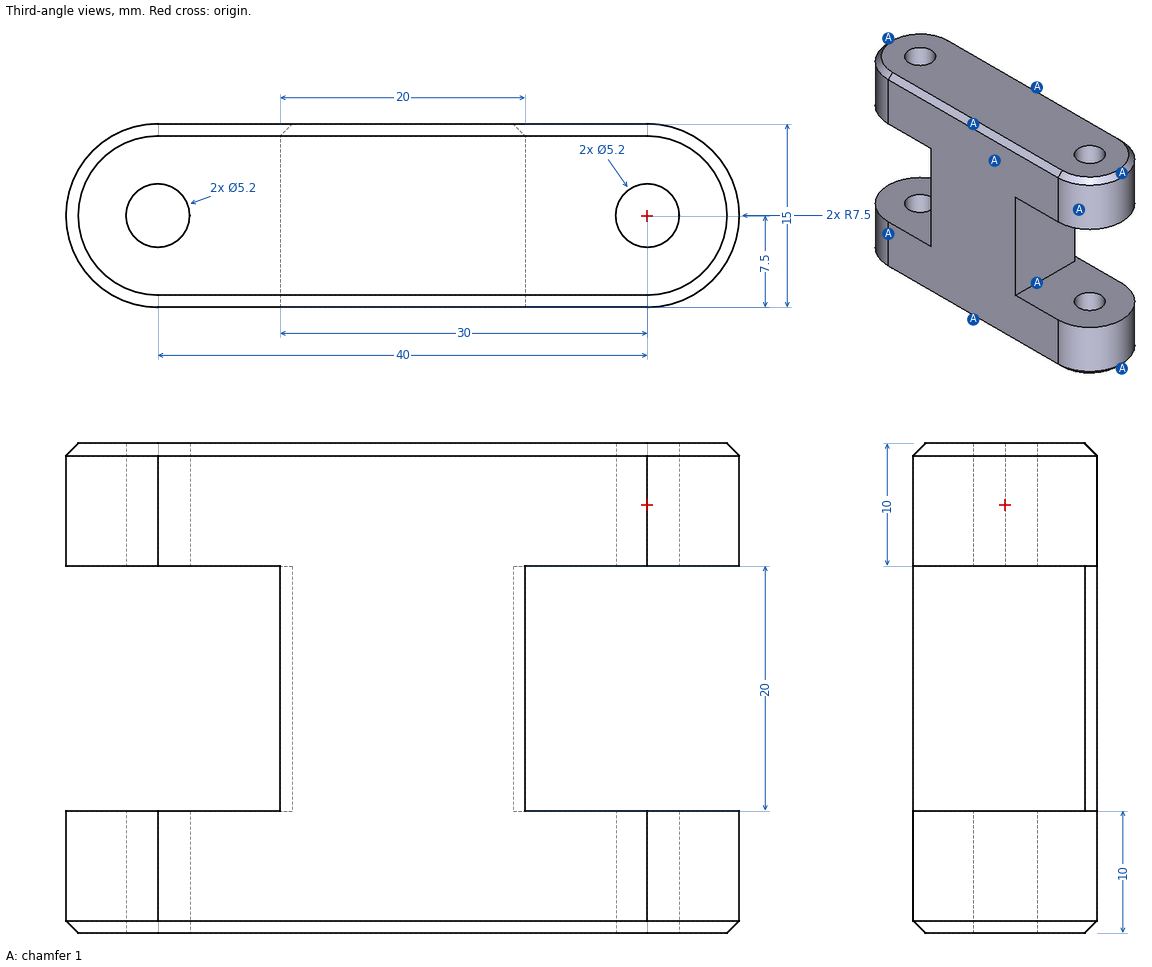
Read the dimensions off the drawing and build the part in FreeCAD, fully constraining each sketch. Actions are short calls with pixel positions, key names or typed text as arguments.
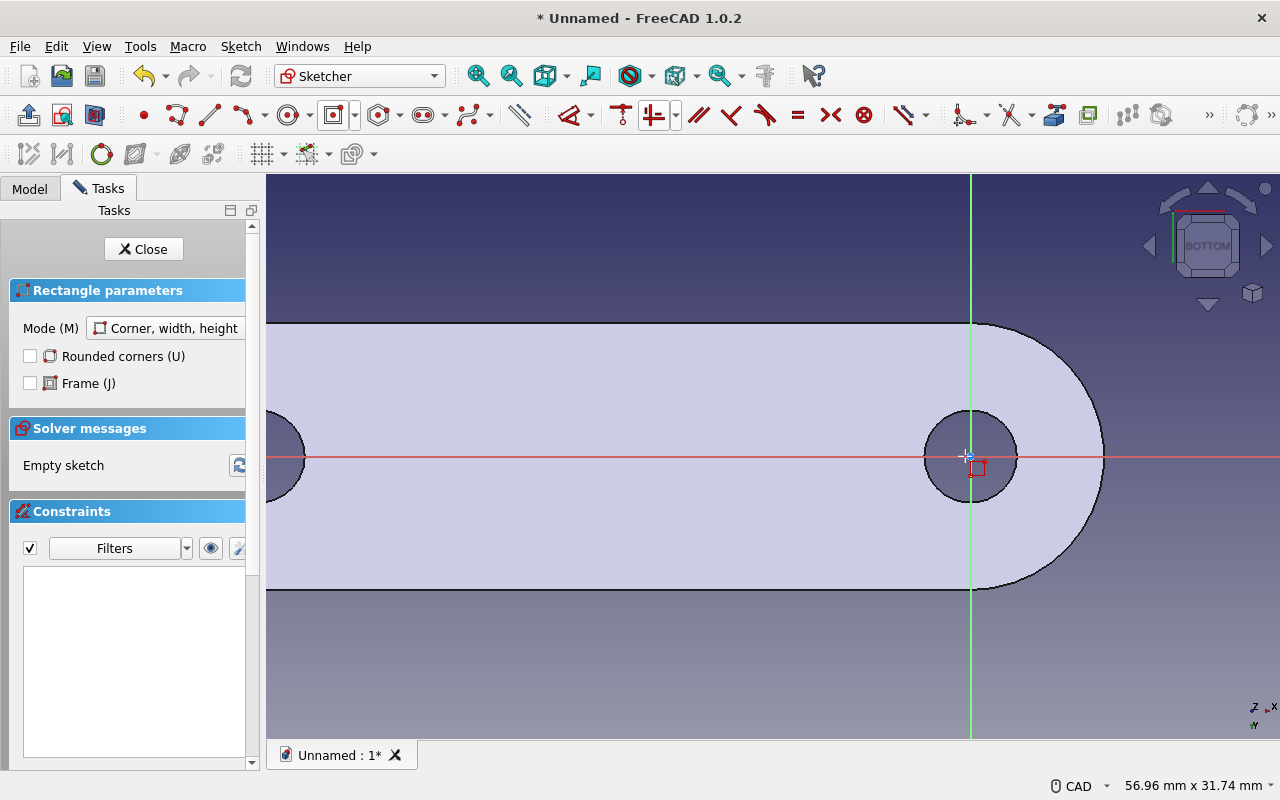
click(437, 323)
move(793, 590)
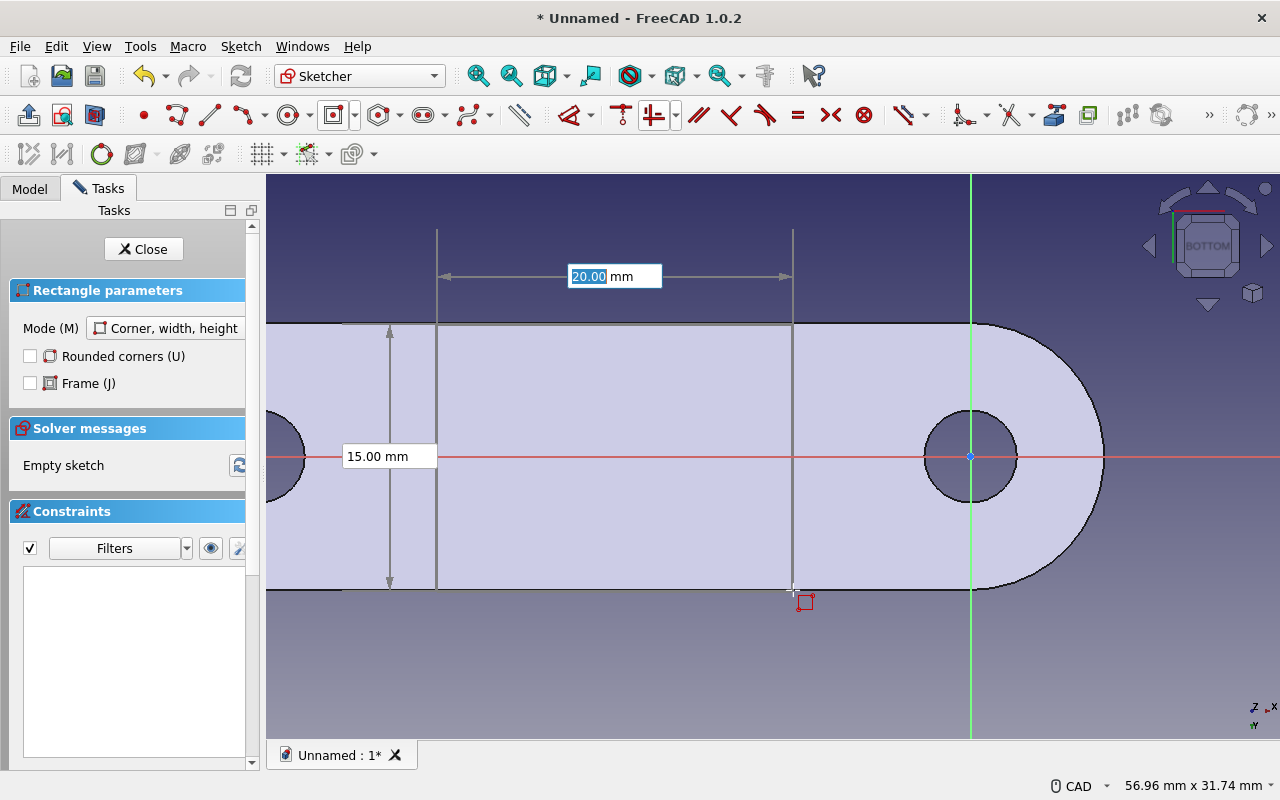
text(20)
key(Tab)
text(15)
key(Return)
key(Escape)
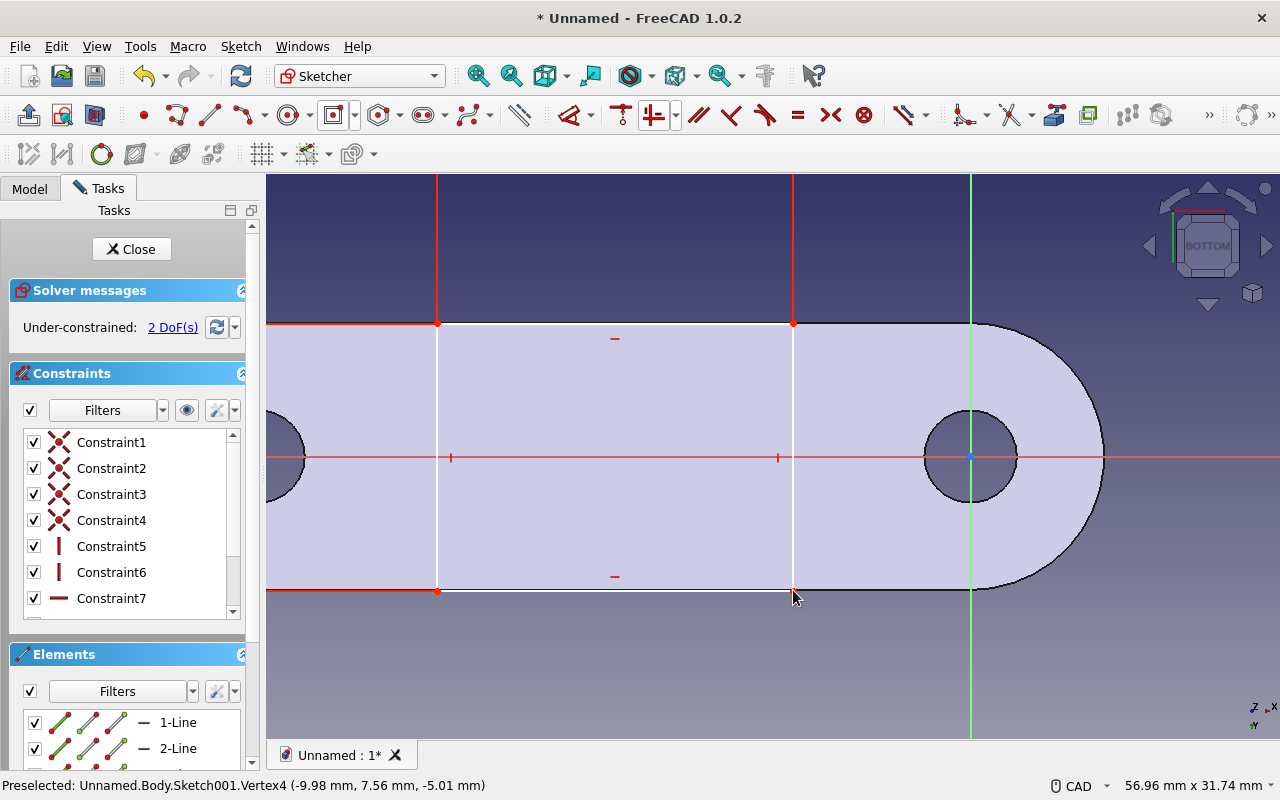
key(d)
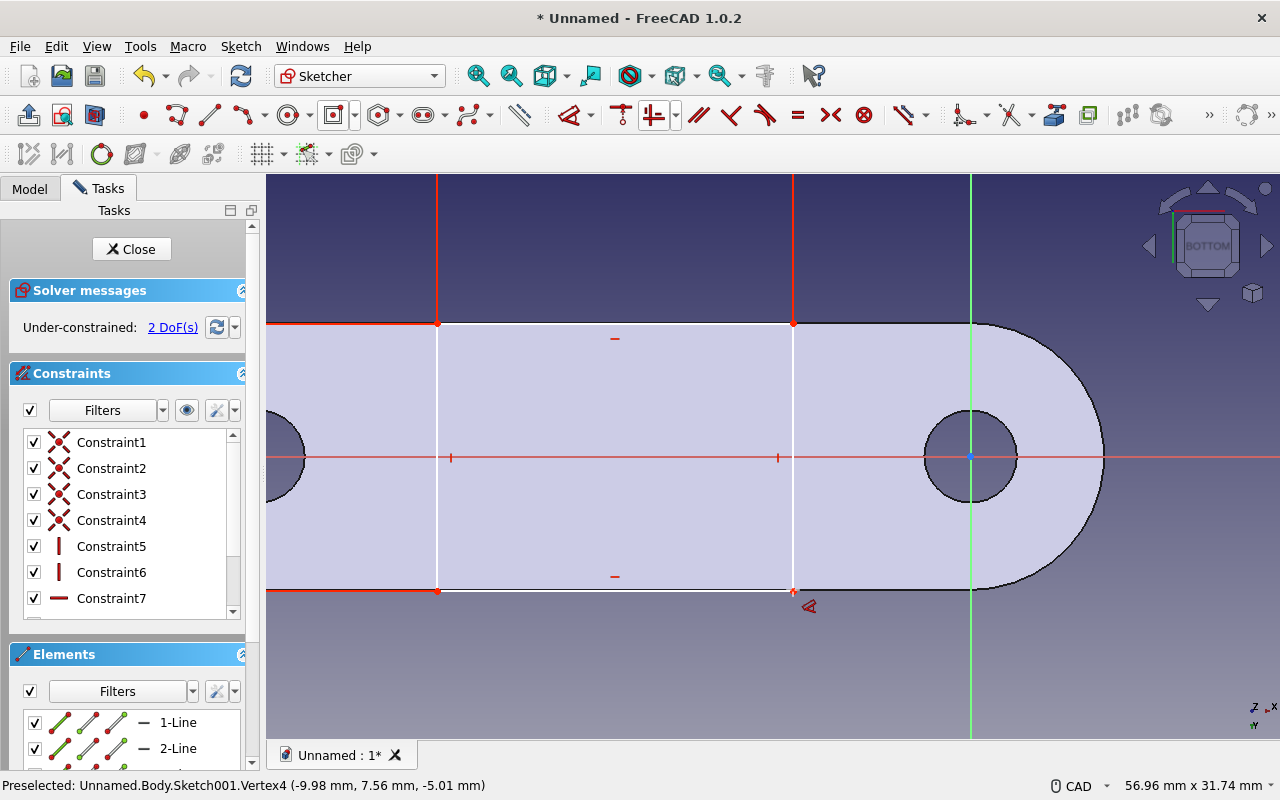
click(437, 324)
click(704, 290)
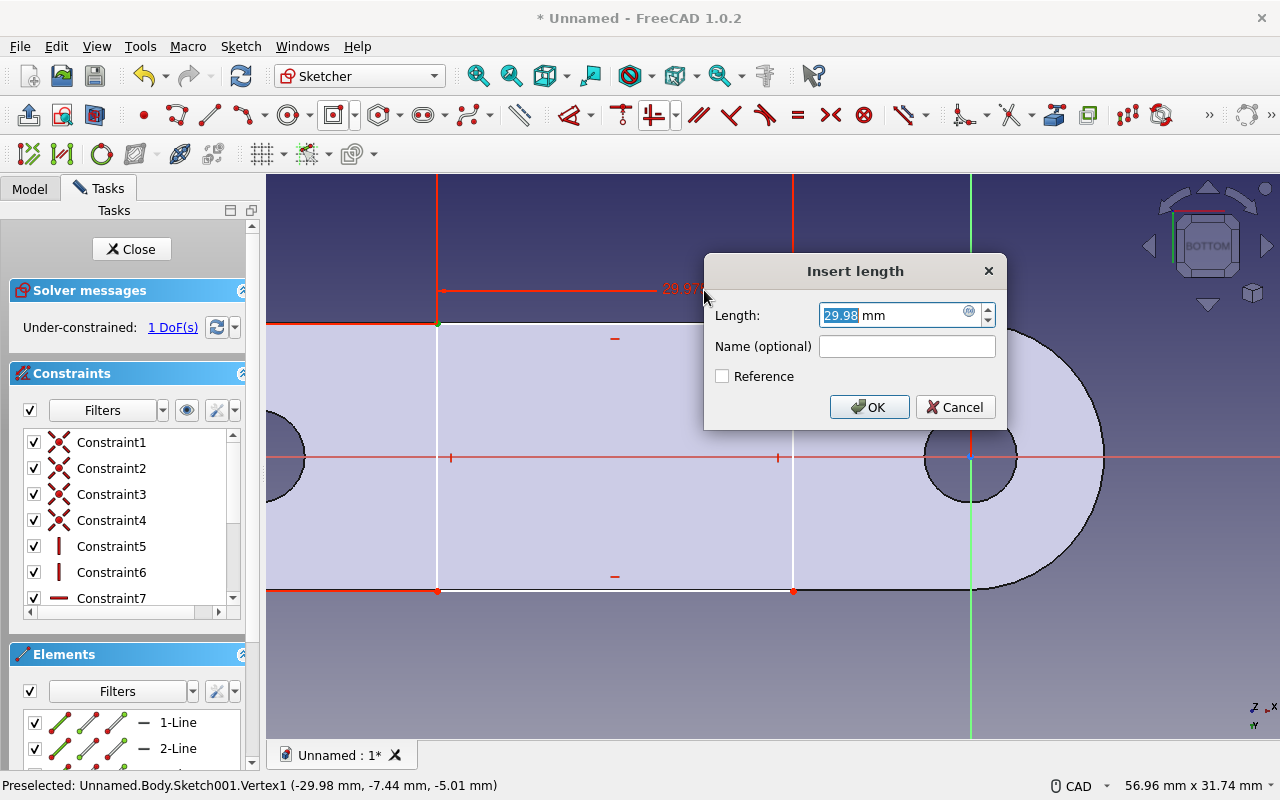
text(30)
key(Return)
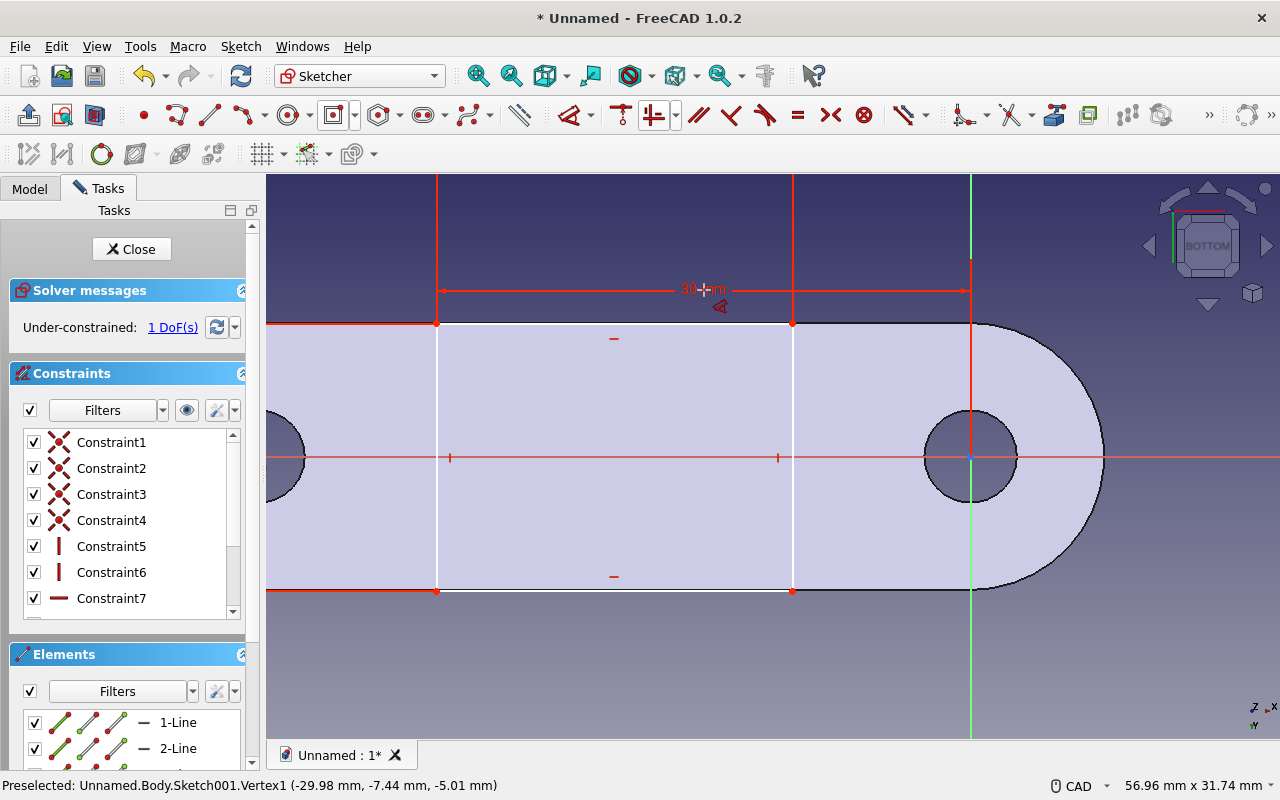
click(437, 324)
click(1005, 390)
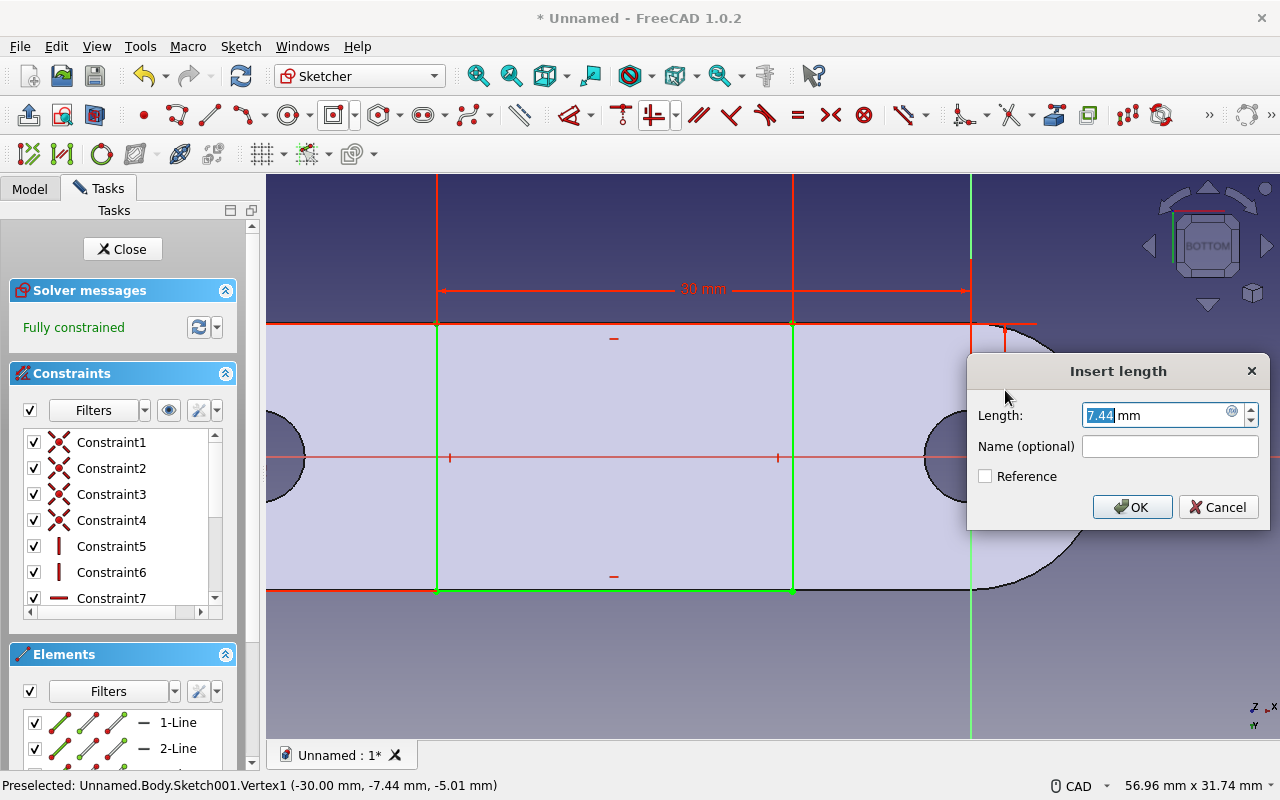
text(7.5)
key(Return)
key(Escape)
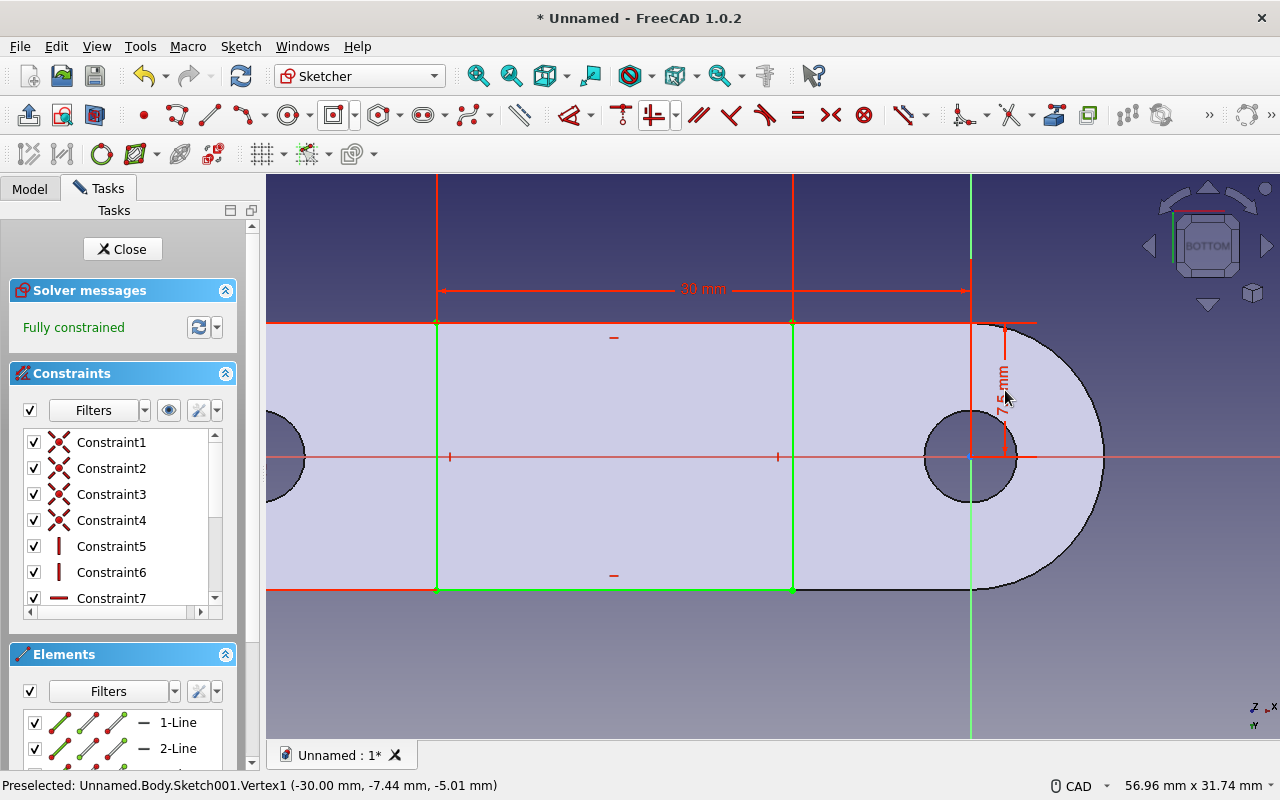
click(123, 249)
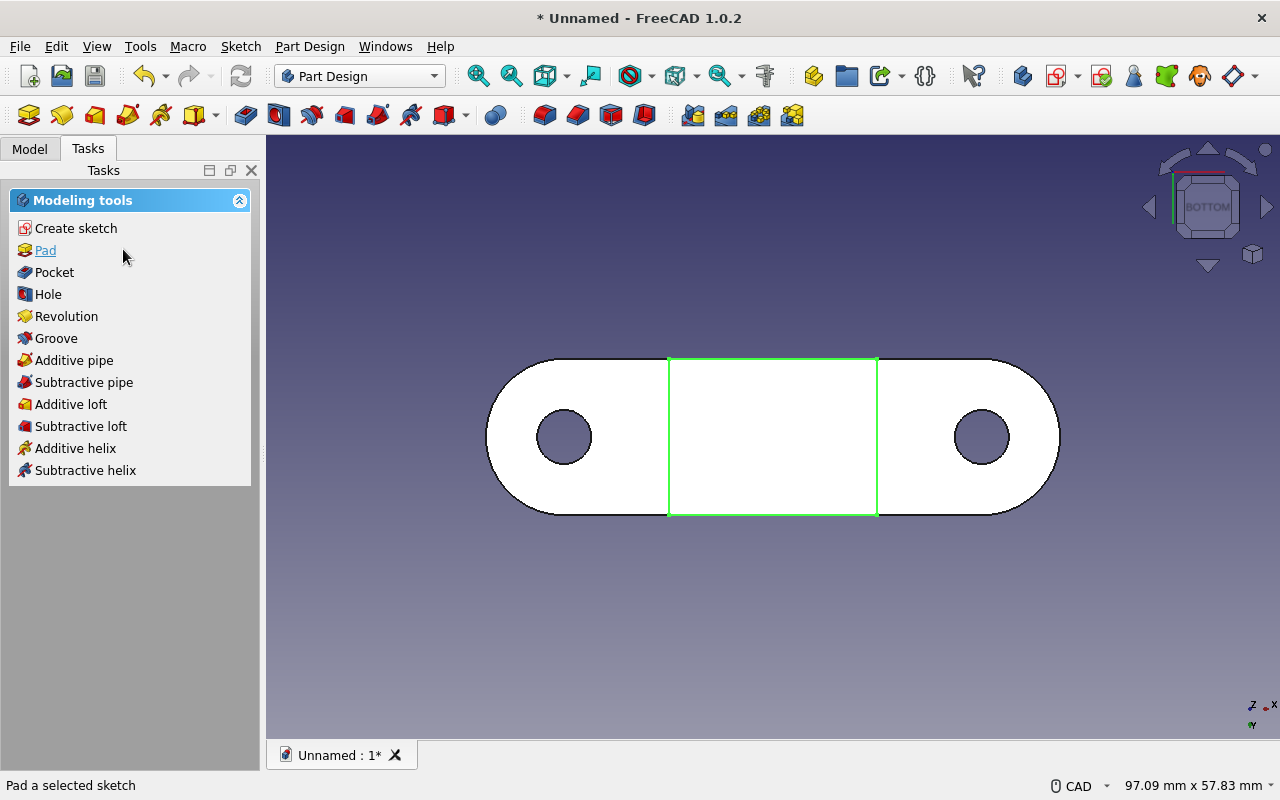
click(29, 116)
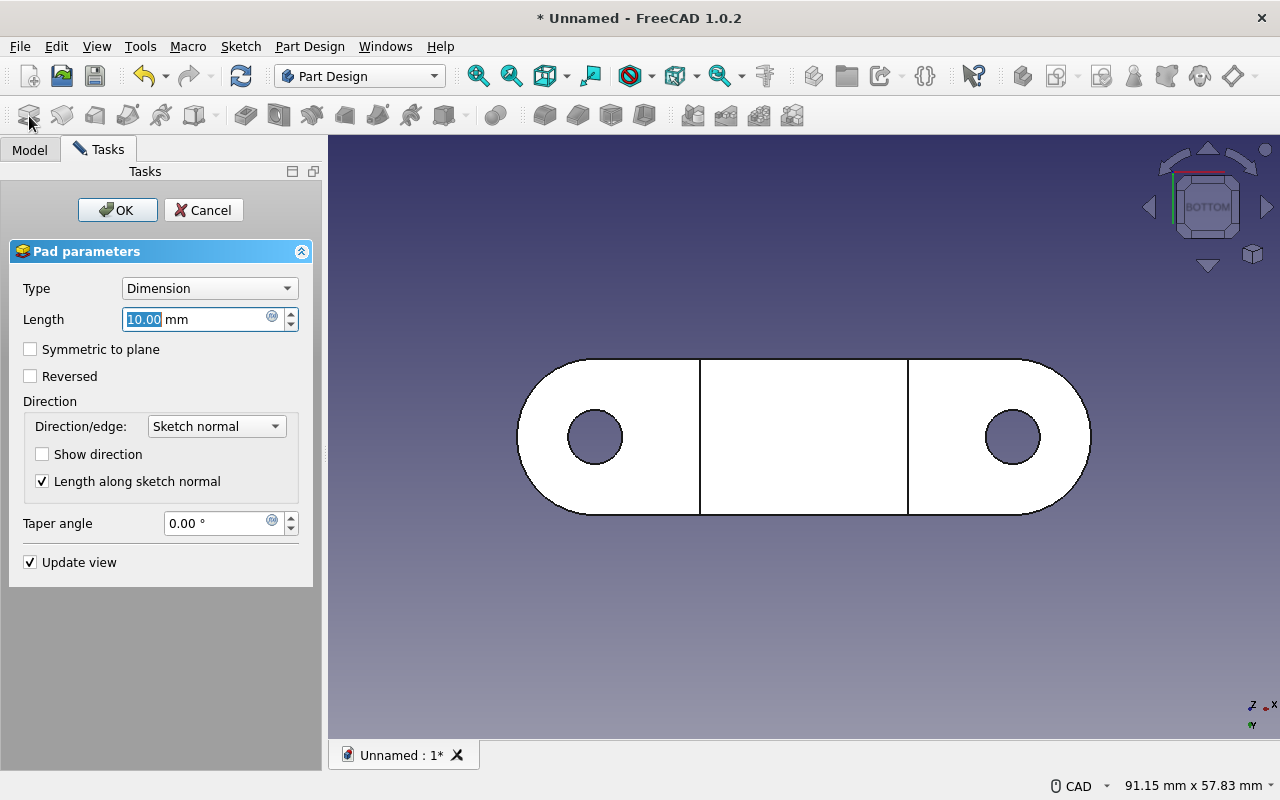
text(20)
key(Tab)